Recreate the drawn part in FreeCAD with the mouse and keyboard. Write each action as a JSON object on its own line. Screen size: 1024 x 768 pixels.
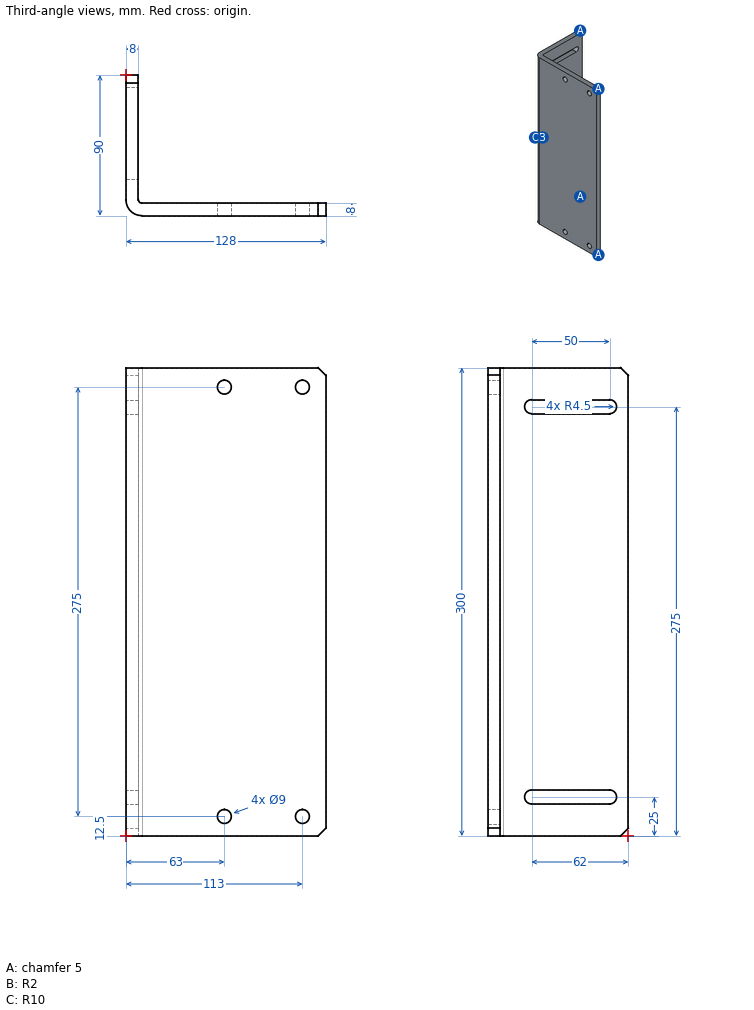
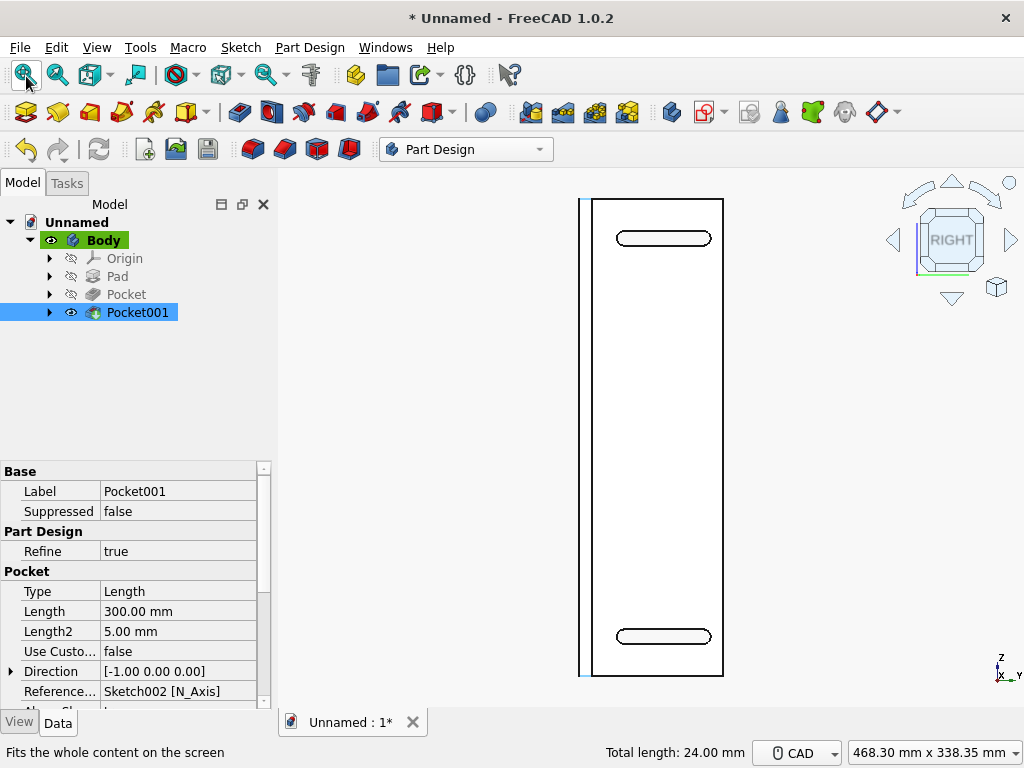
{"action": "key", "text": "5"}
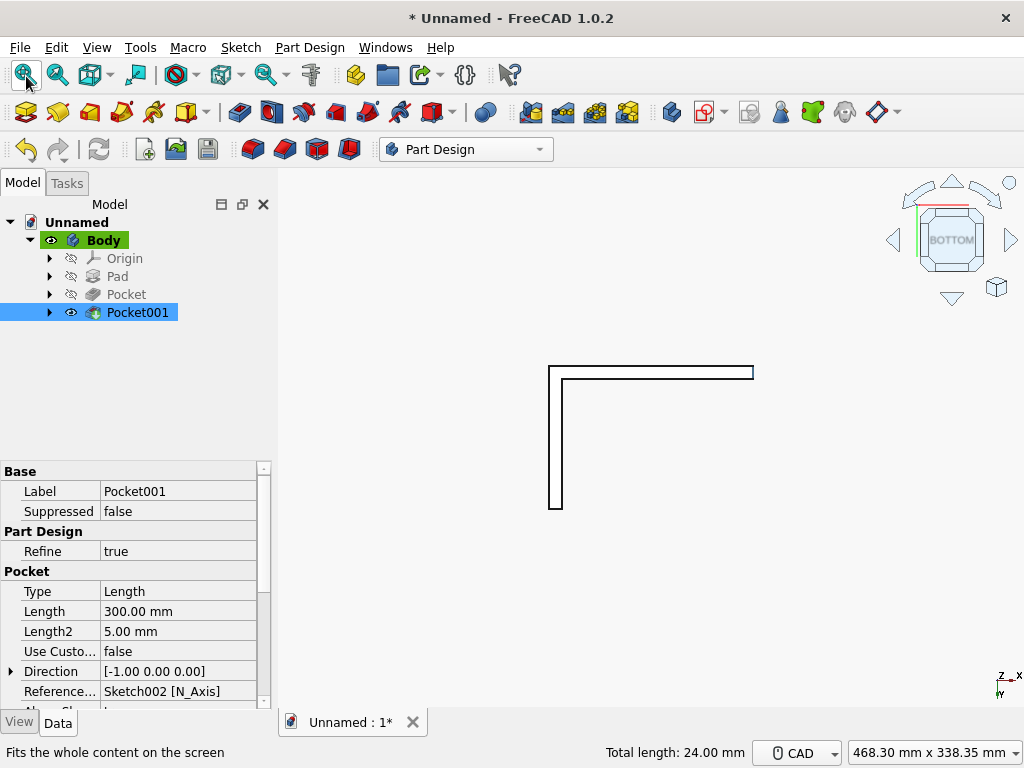
{"action": "left_click", "coordinate": [26, 76]}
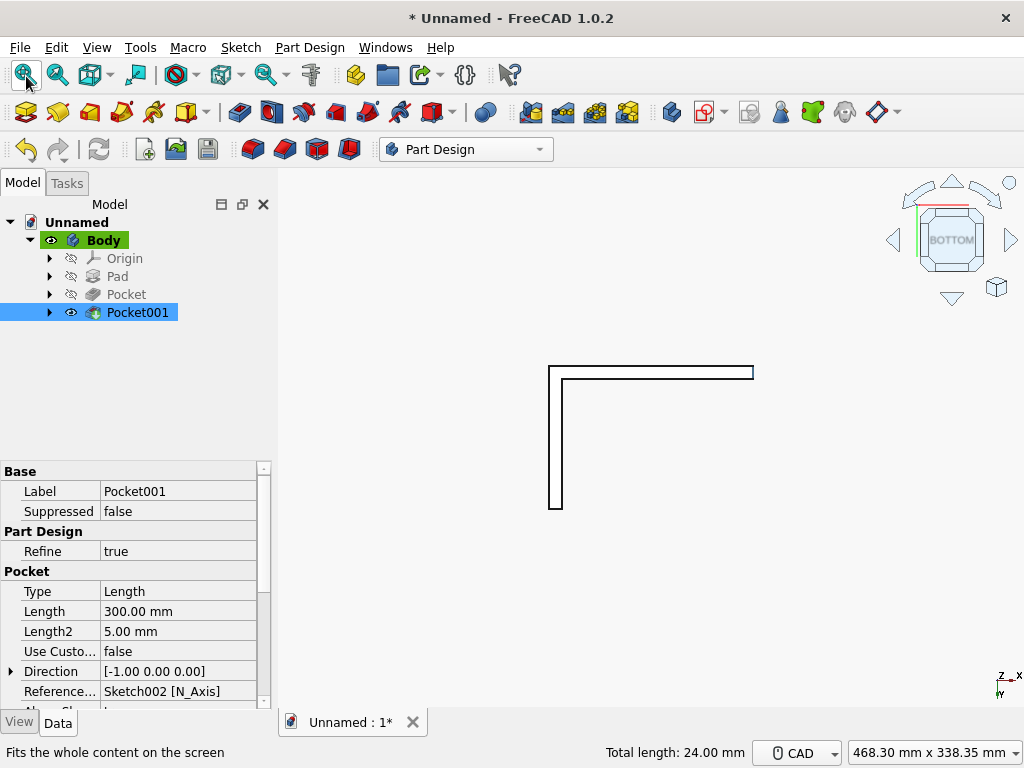
{"action": "scroll", "coordinate": [555, 508], "scroll_direction": "up", "scroll_amount": 6}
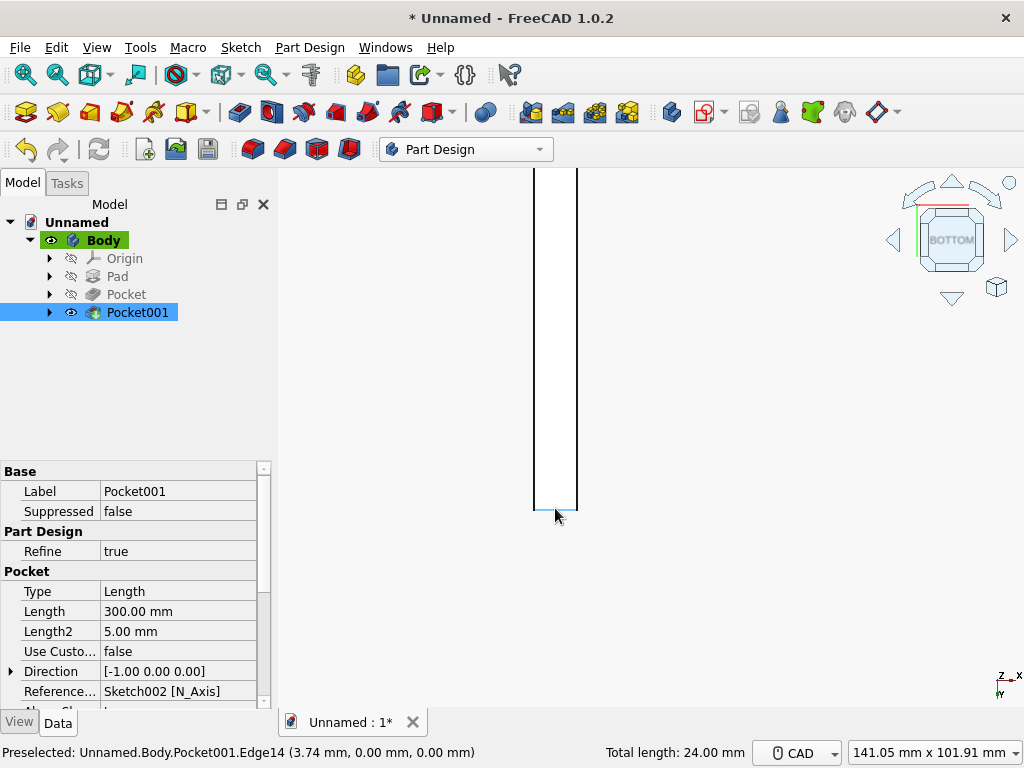
{"action": "left_click", "coordinate": [556, 509], "text": "ctrl"}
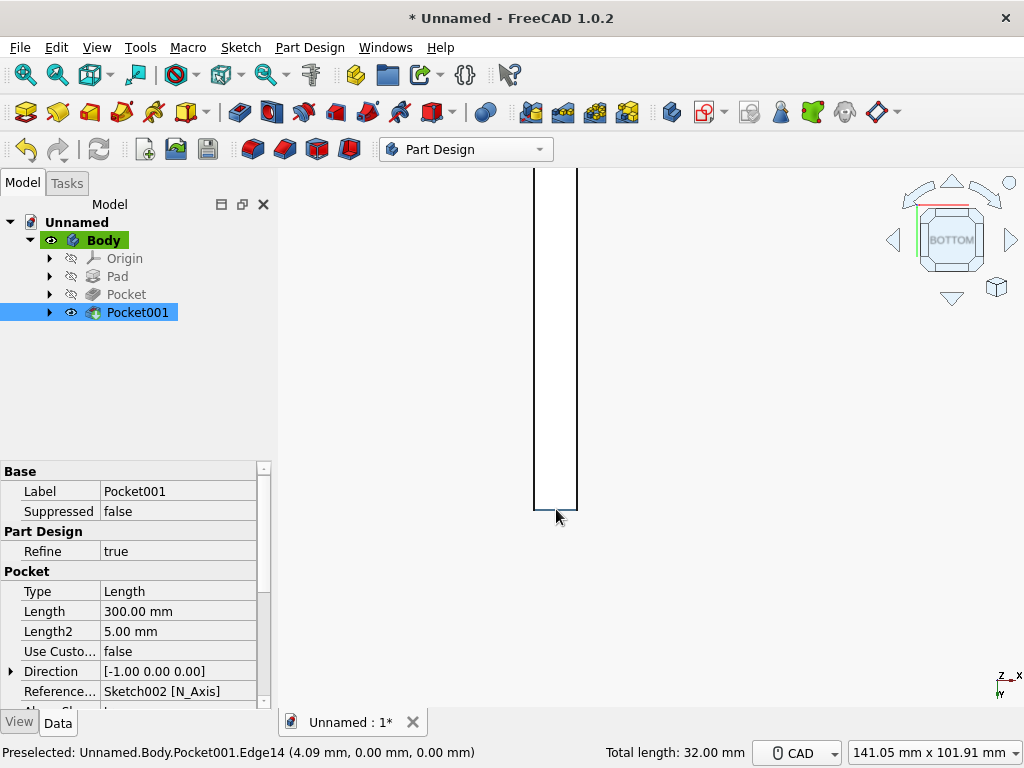
{"action": "left_click", "coordinate": [286, 150]}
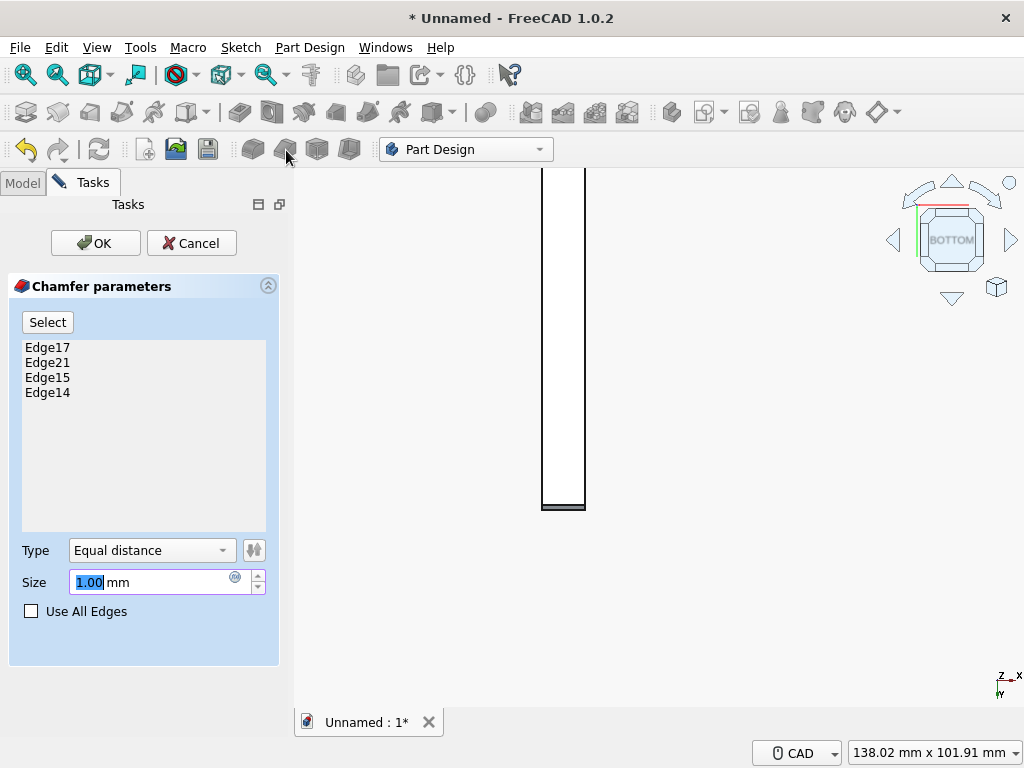
{"action": "type", "text": "5"}
{"action": "key", "text": "Tab"}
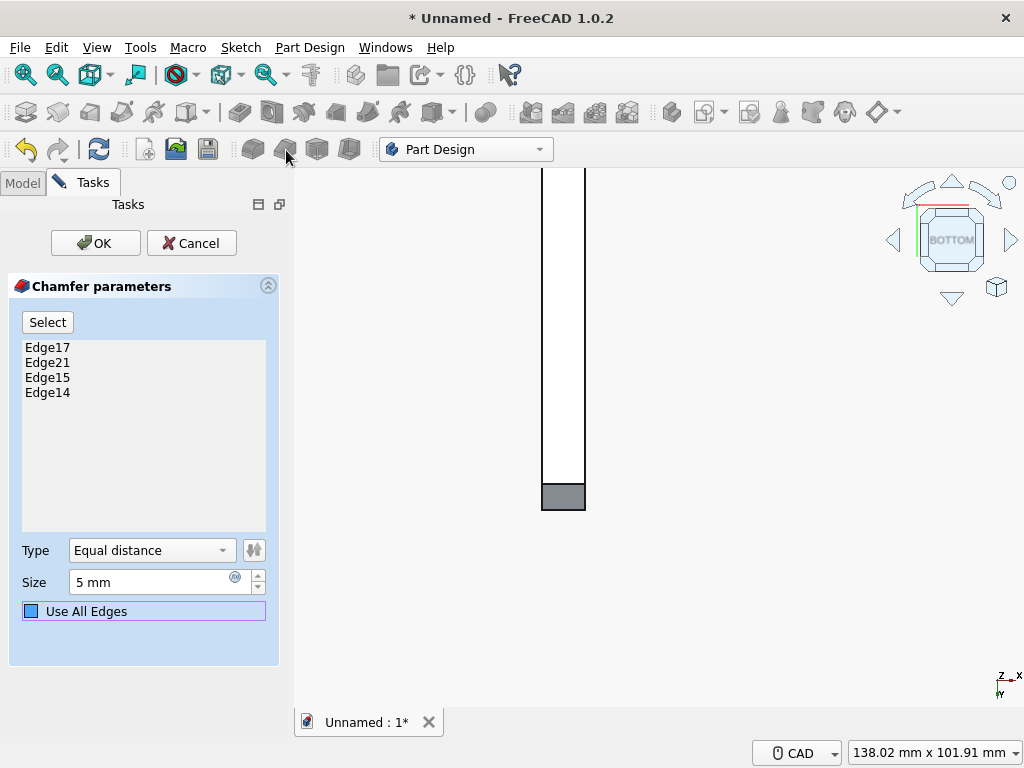
{"action": "left_click", "coordinate": [96, 243]}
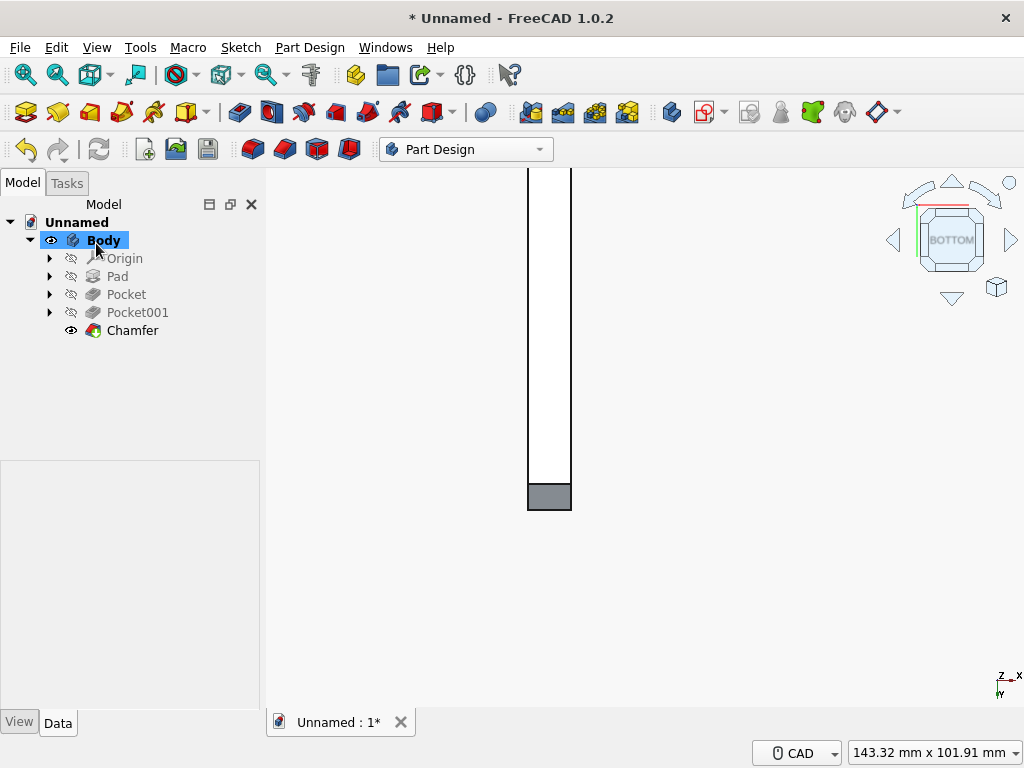
{"action": "key", "text": "v f"}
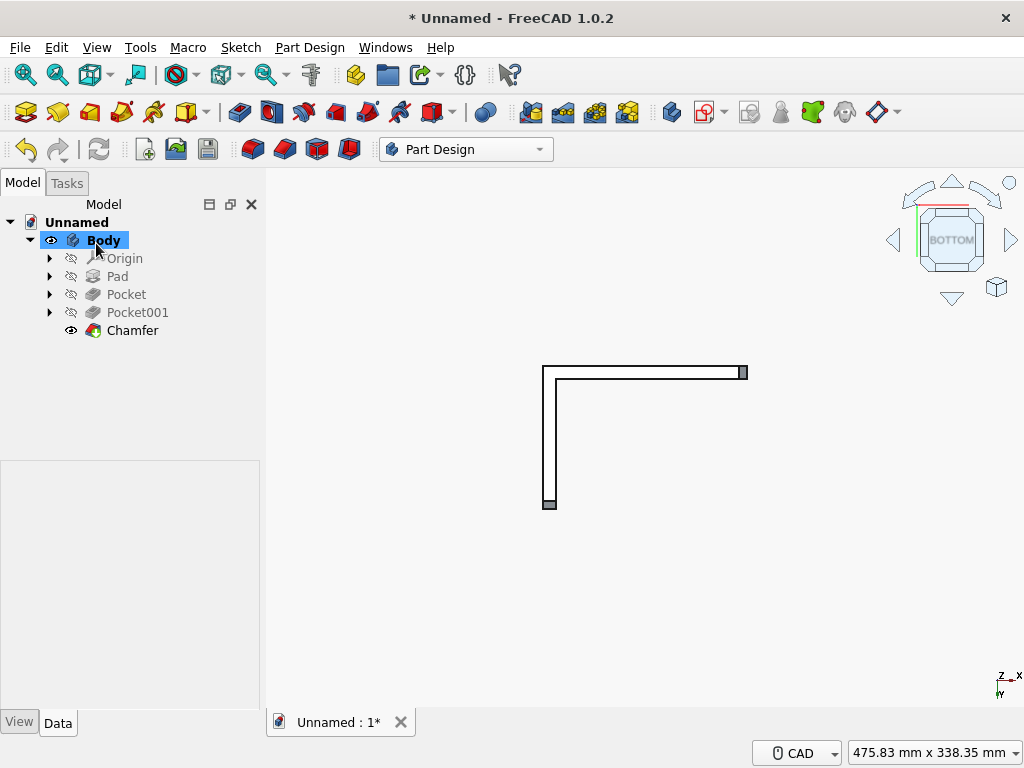
{"action": "key", "text": "0"}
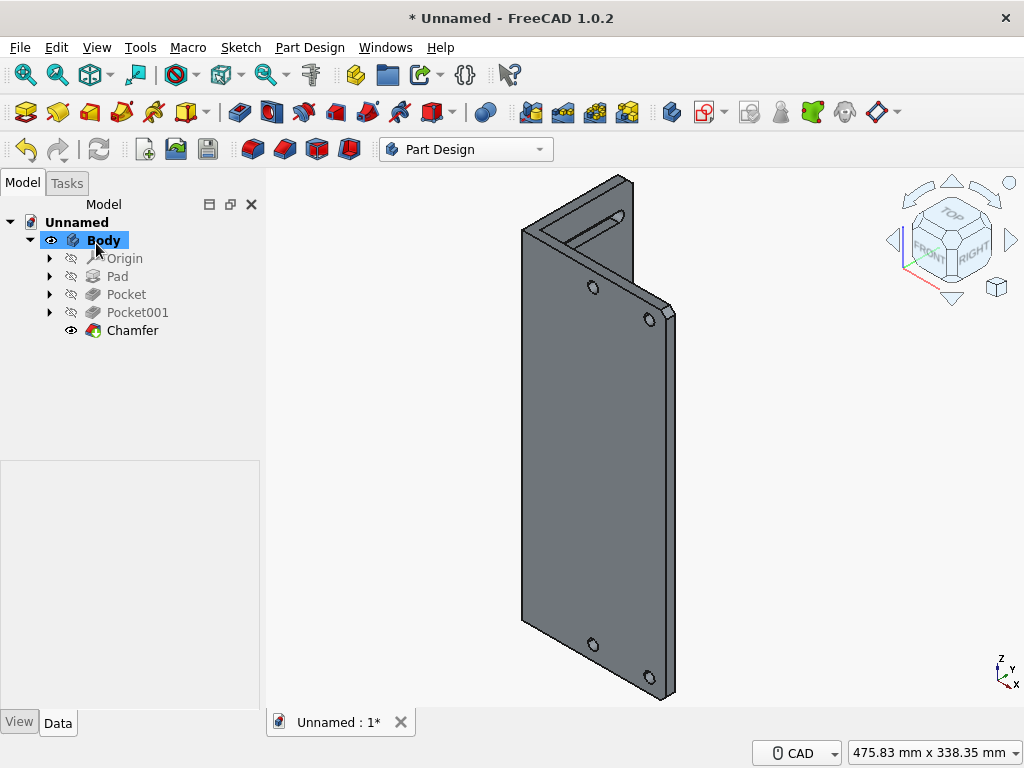
{"action": "key", "text": "2"}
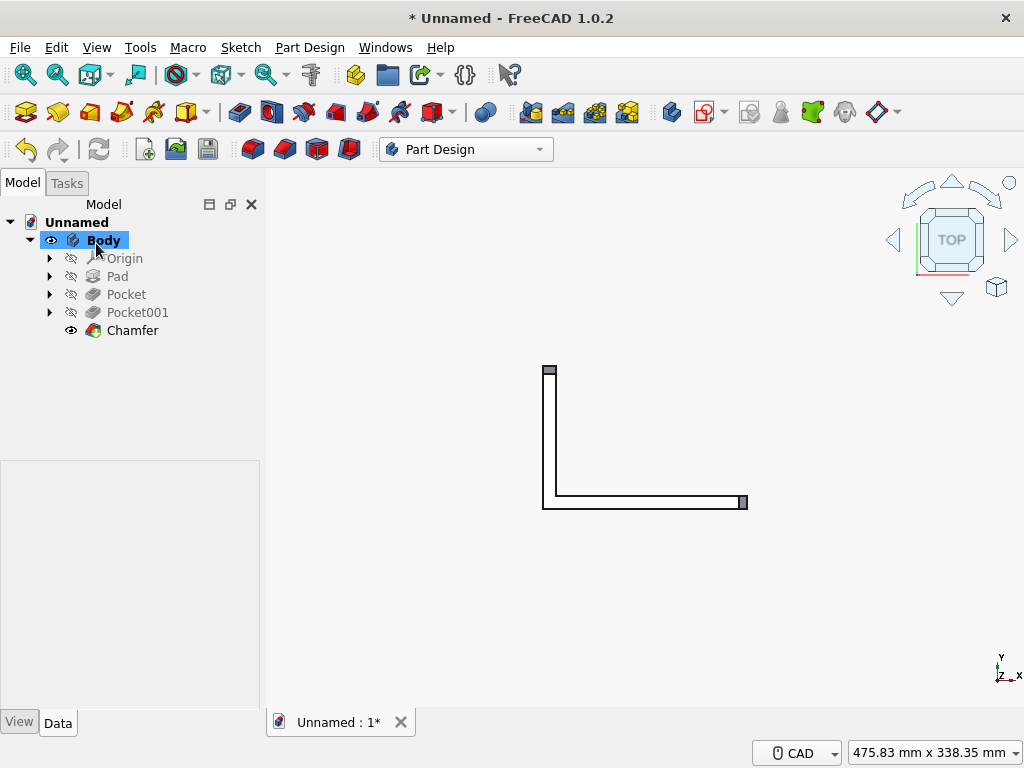
{"action": "left_click", "coordinate": [26, 76]}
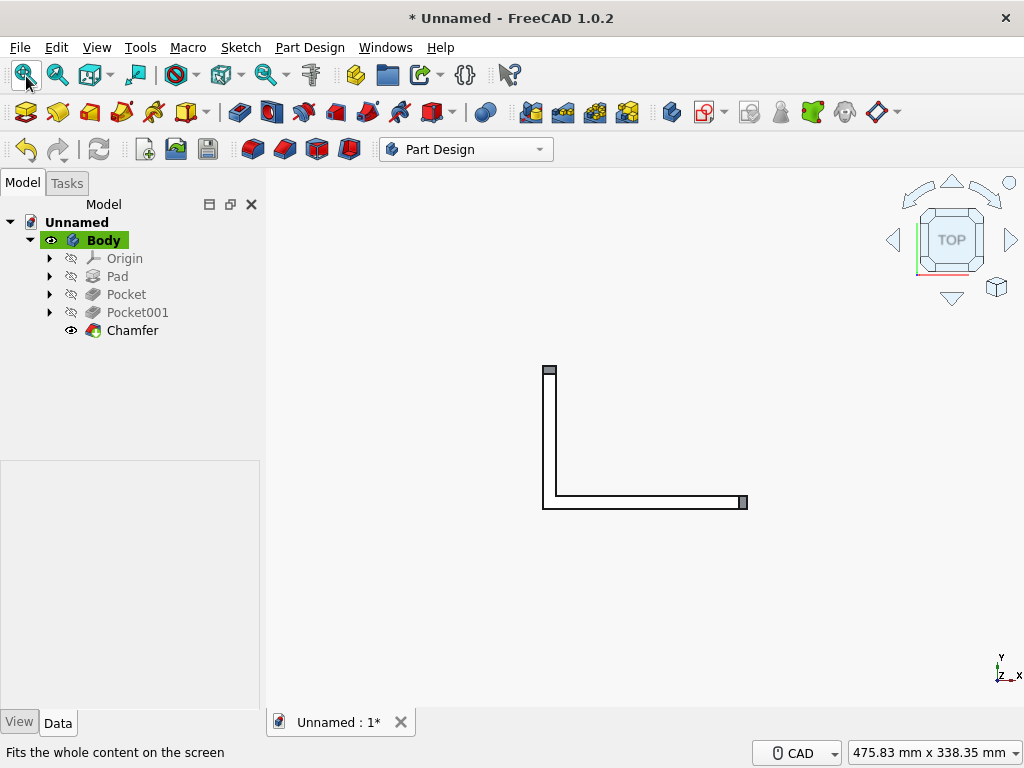
{"action": "key", "text": "1"}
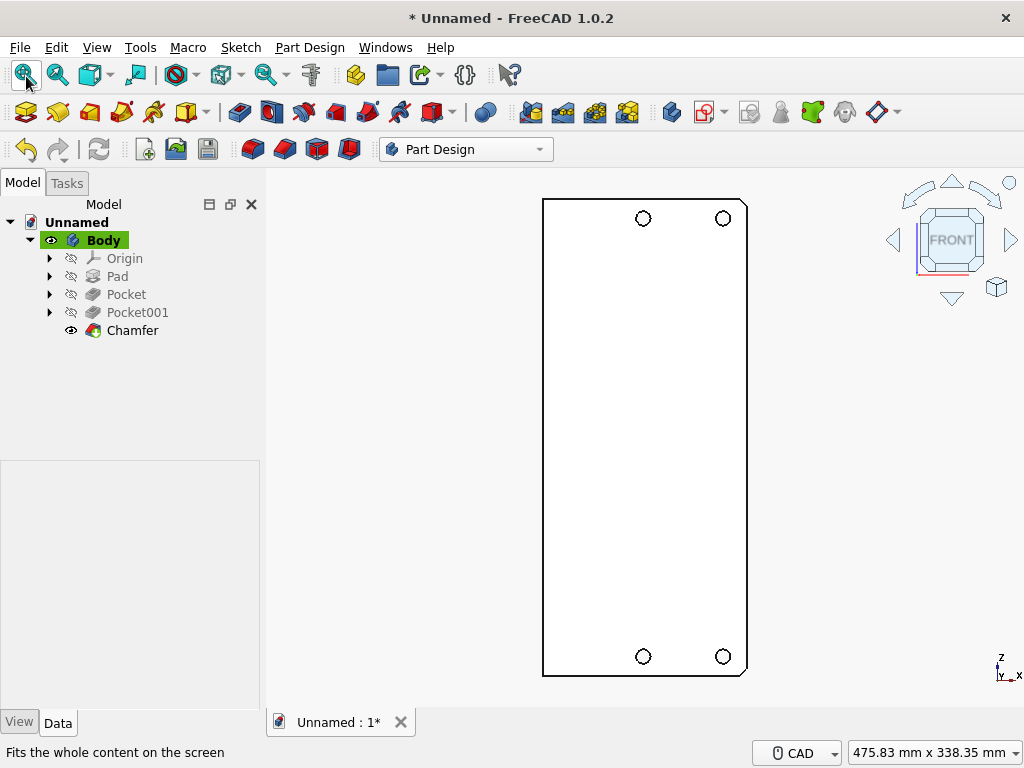
{"action": "key", "text": "3"}